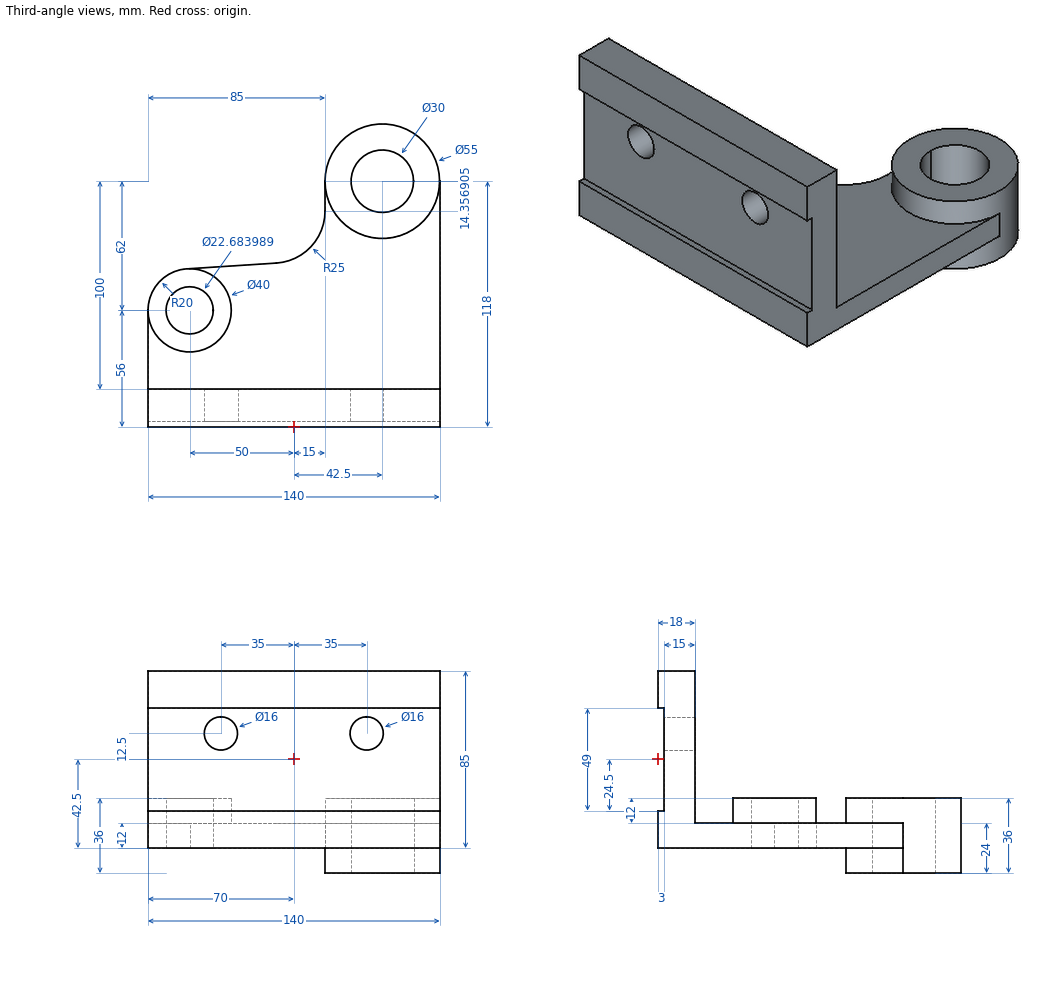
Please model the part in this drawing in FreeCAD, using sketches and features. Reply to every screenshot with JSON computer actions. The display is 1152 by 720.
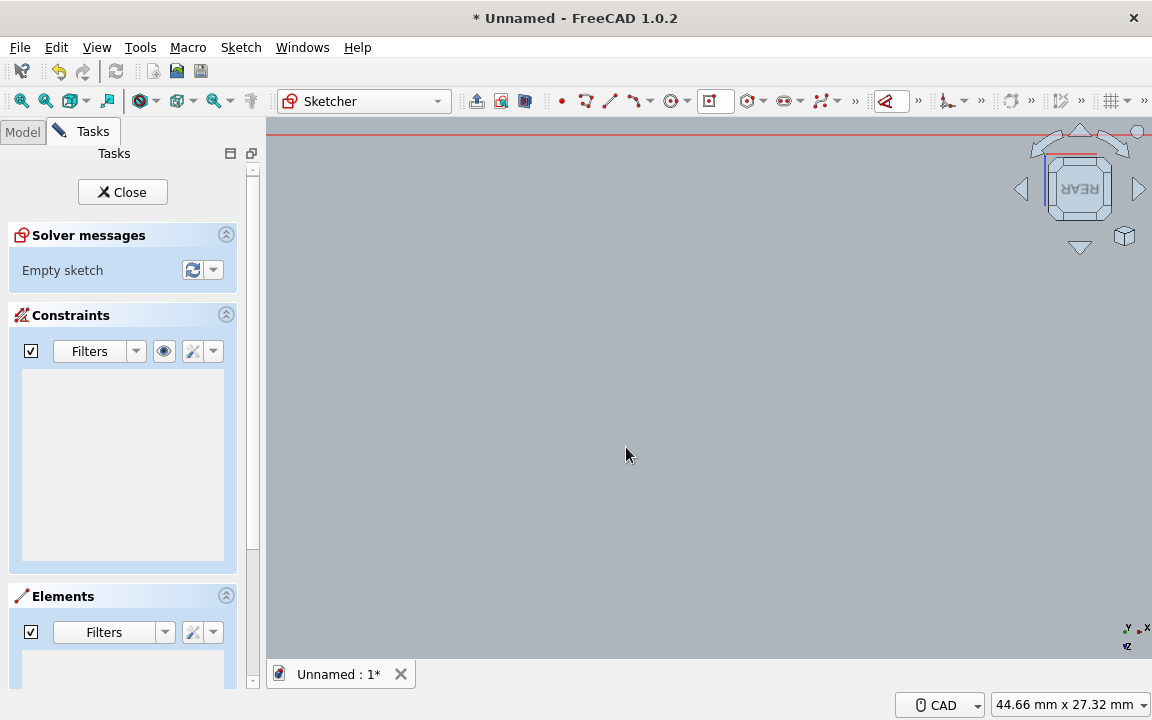
{"action": "key", "text": "g c"}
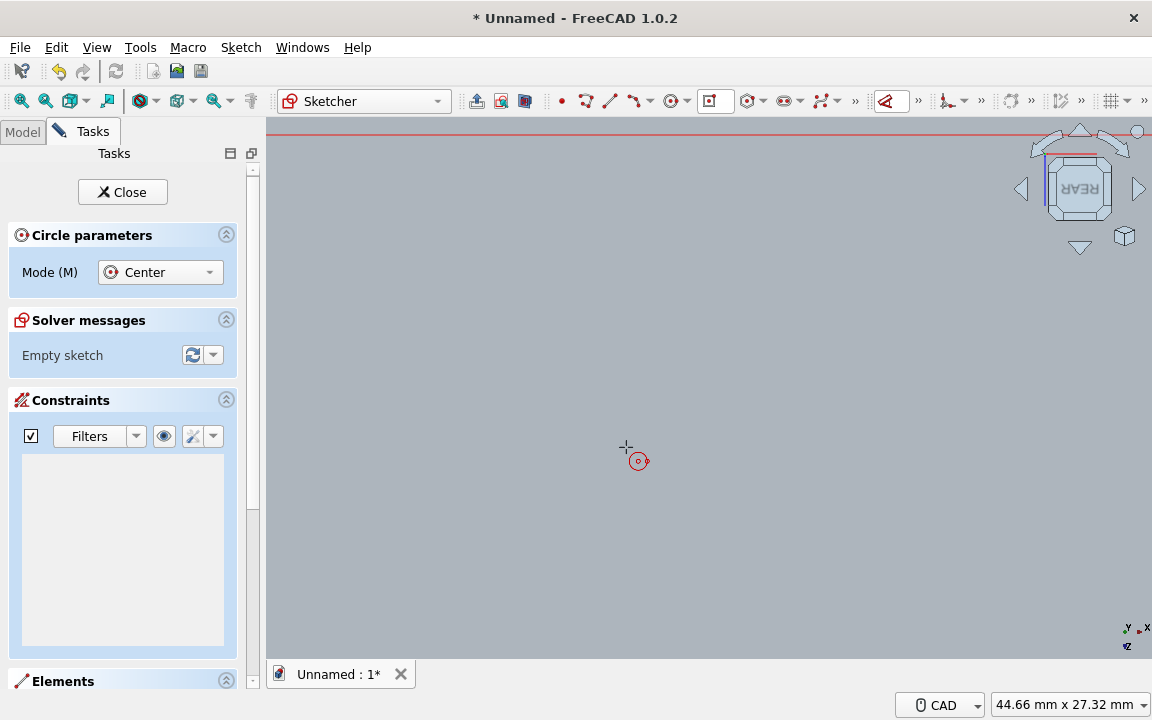
{"action": "left_click", "coordinate": [640, 383]}
{"action": "left_click", "coordinate": [753, 271]}
{"action": "key", "text": "Escape"}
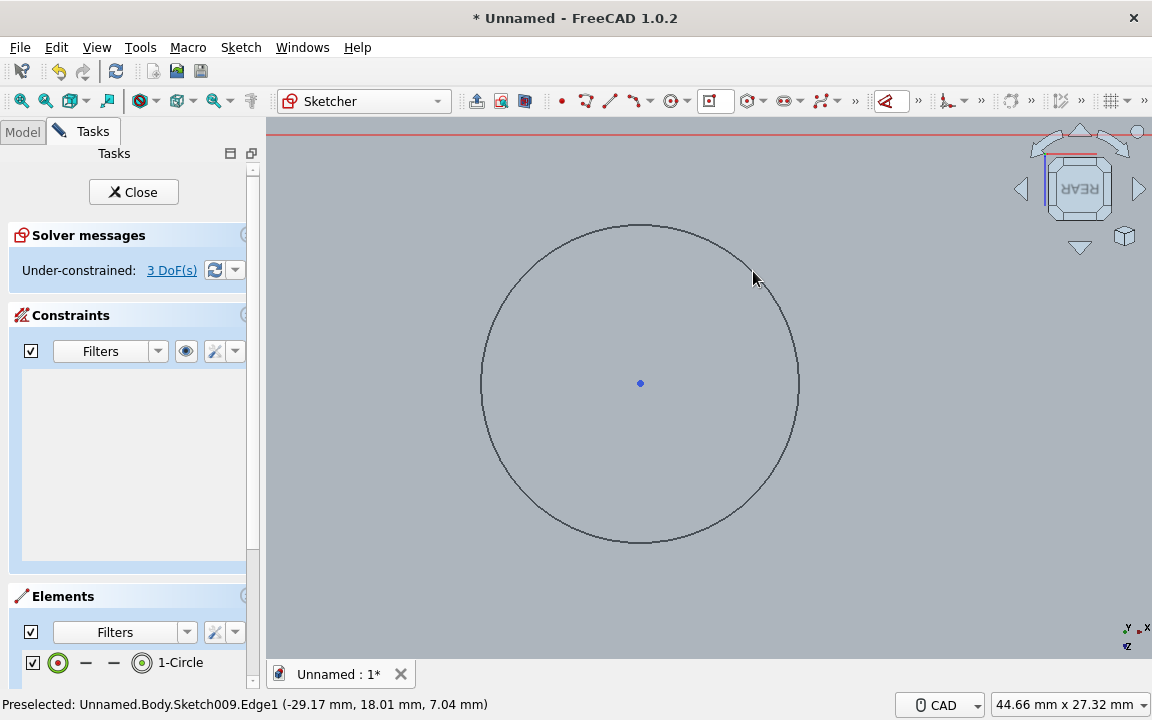
{"action": "left_click", "coordinate": [752, 271]}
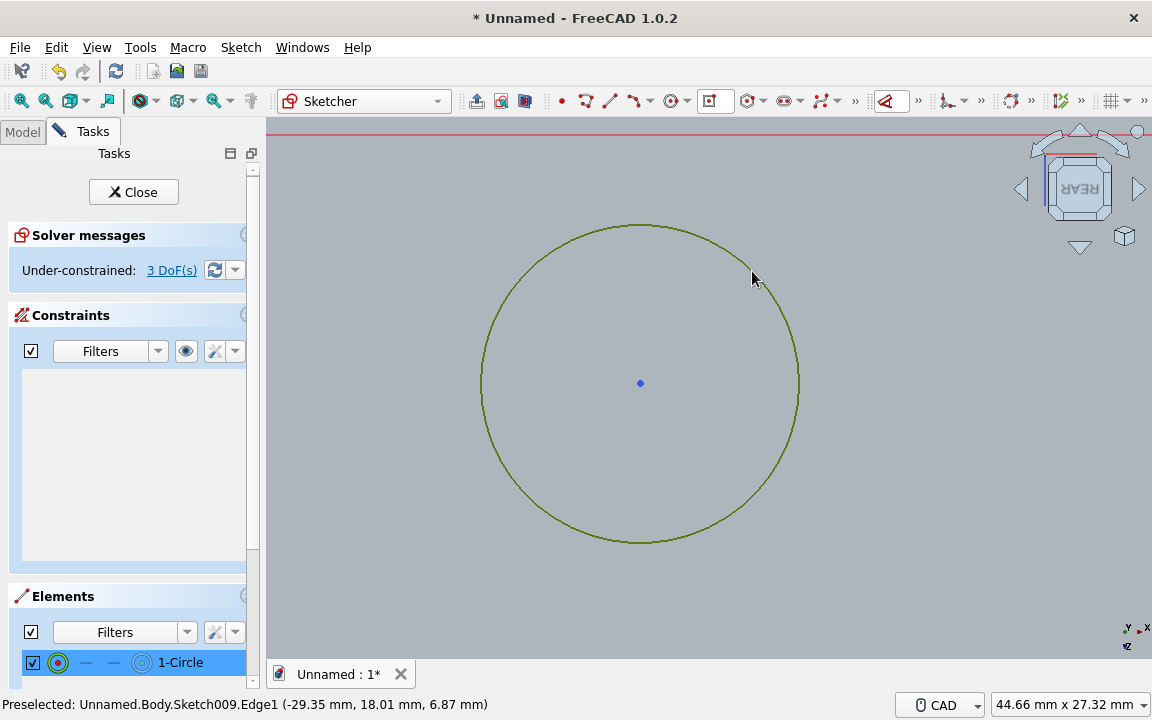
{"action": "key", "text": "k o"}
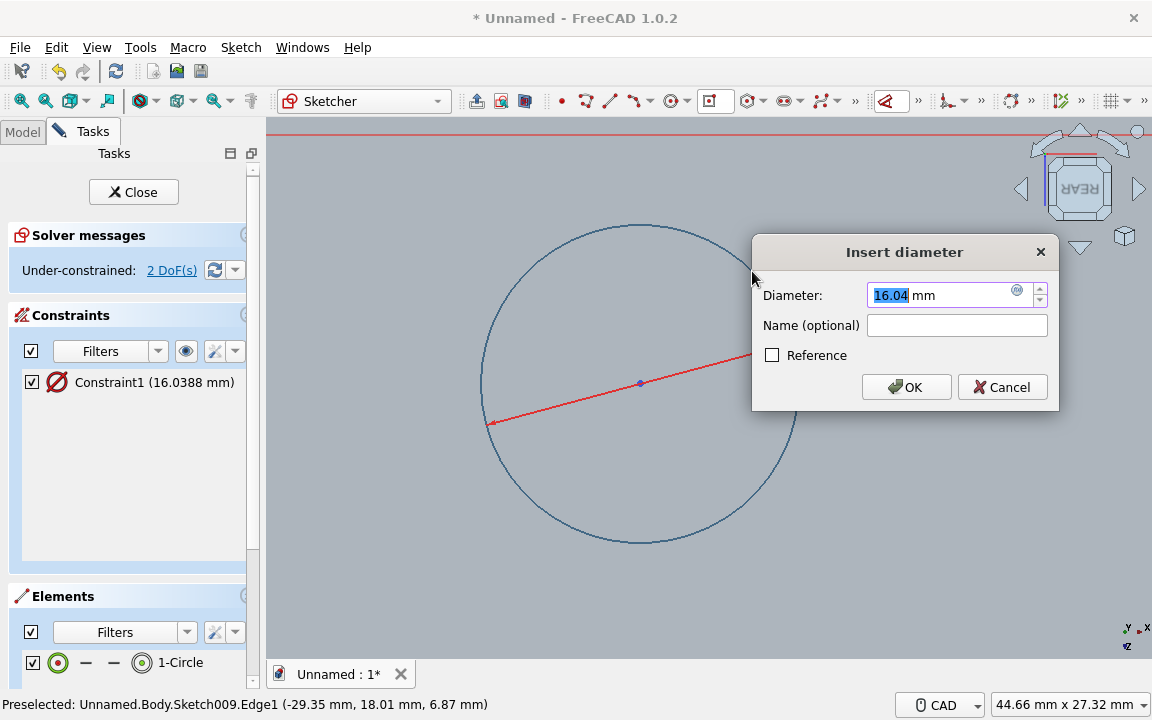
{"action": "type", "text": "16"}
{"action": "key", "text": "Return"}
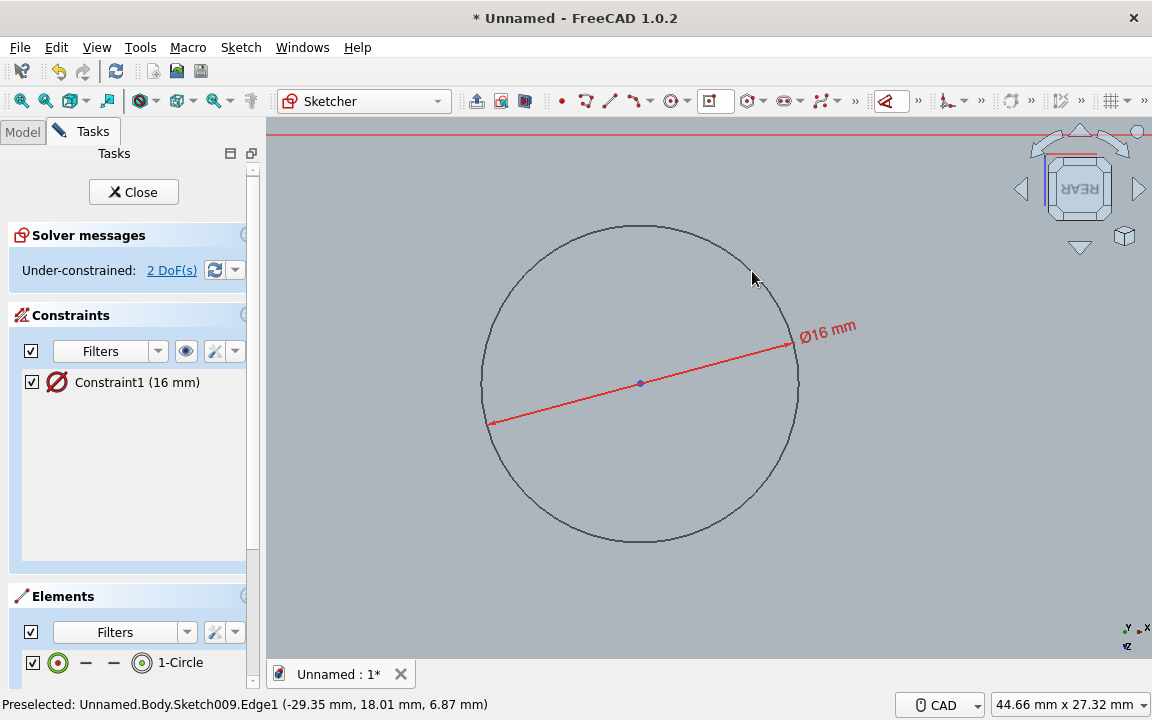
{"action": "left_click", "coordinate": [640, 384]}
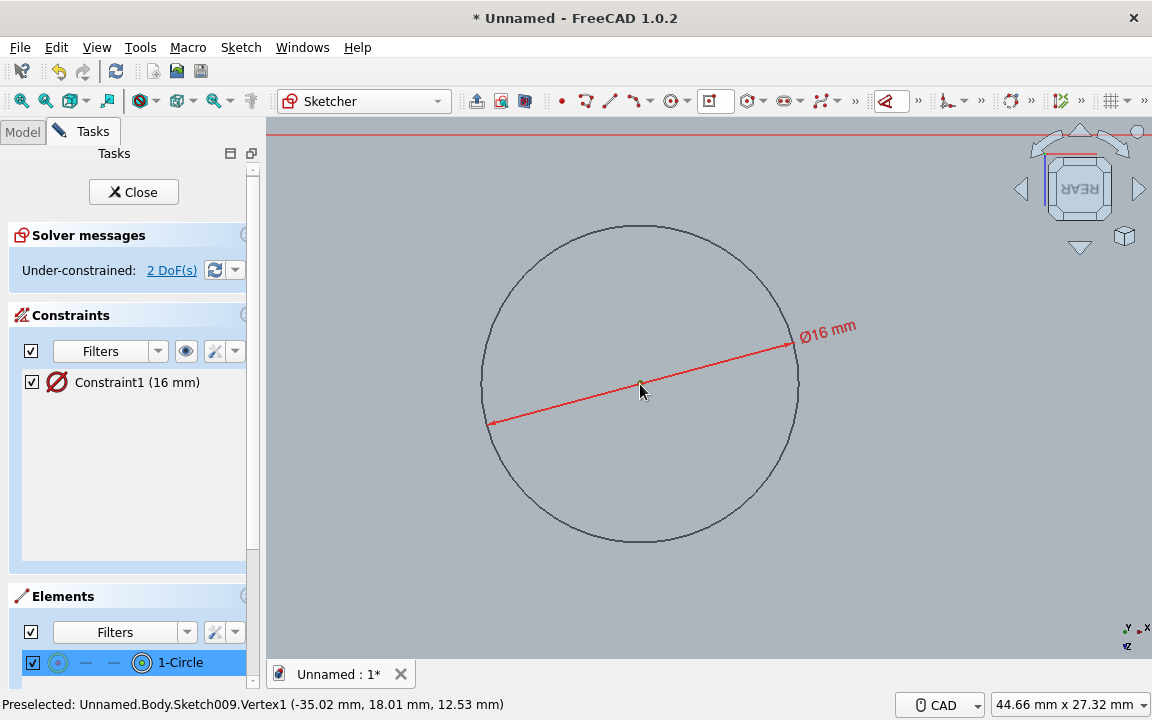
{"action": "key", "text": "l"}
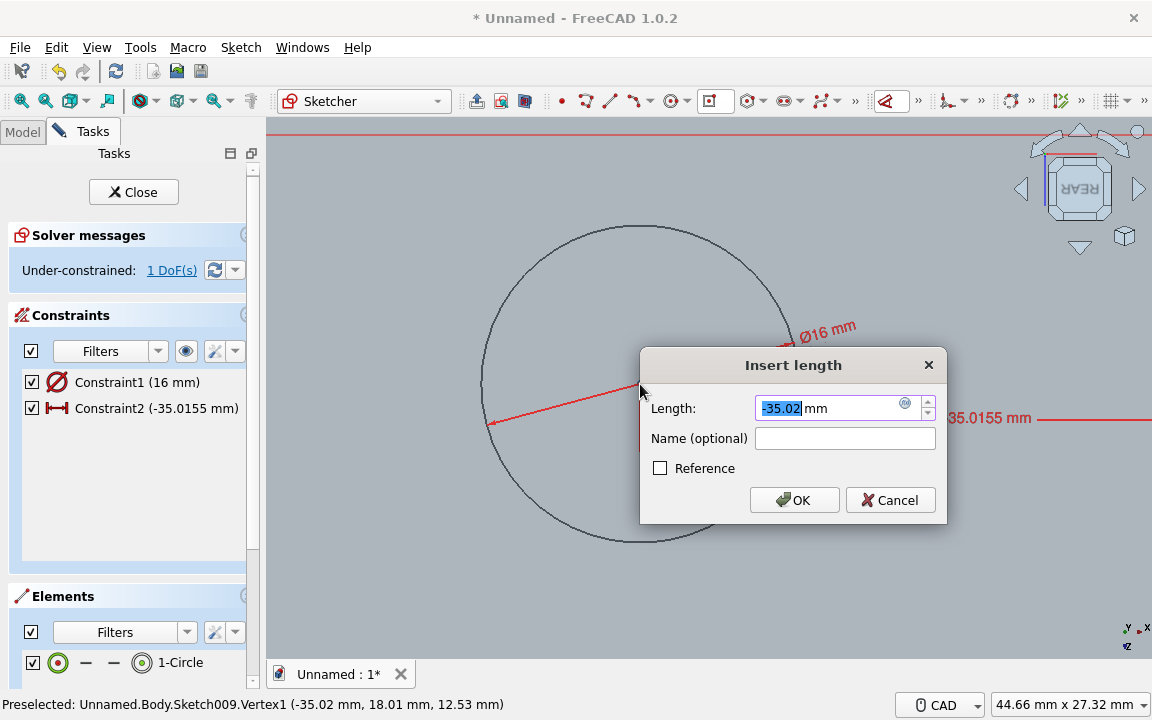
{"action": "type", "text": "-35"}
{"action": "key", "text": "Return"}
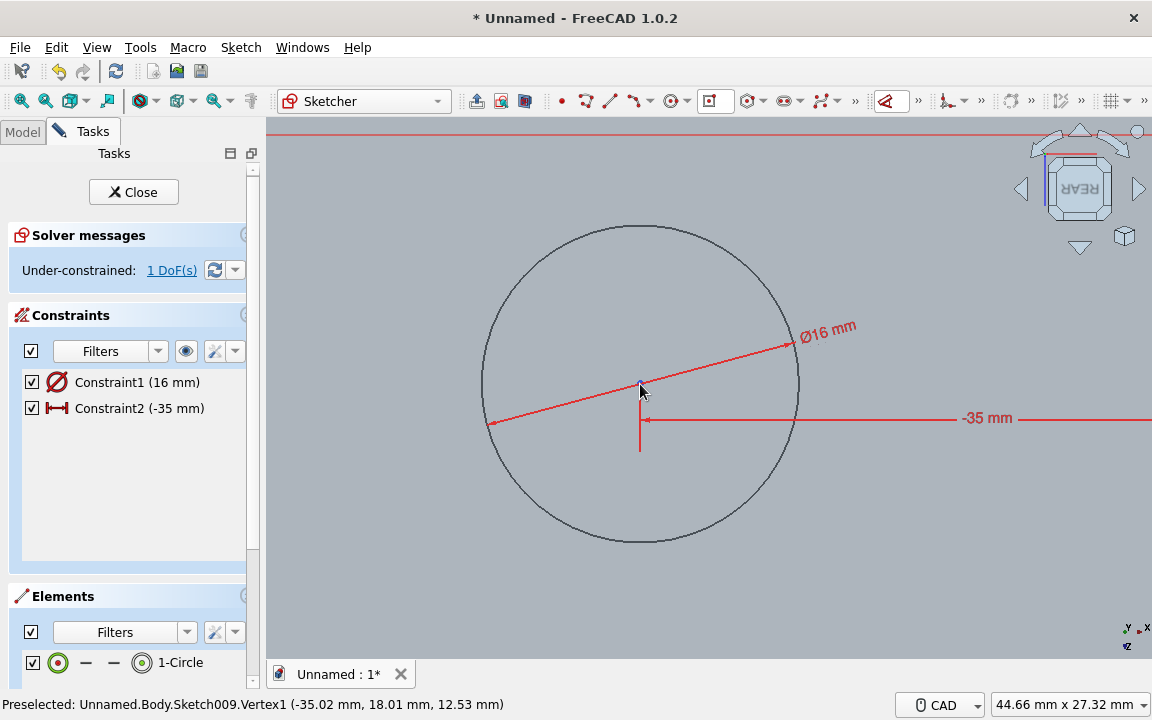
{"action": "left_click", "coordinate": [640, 384]}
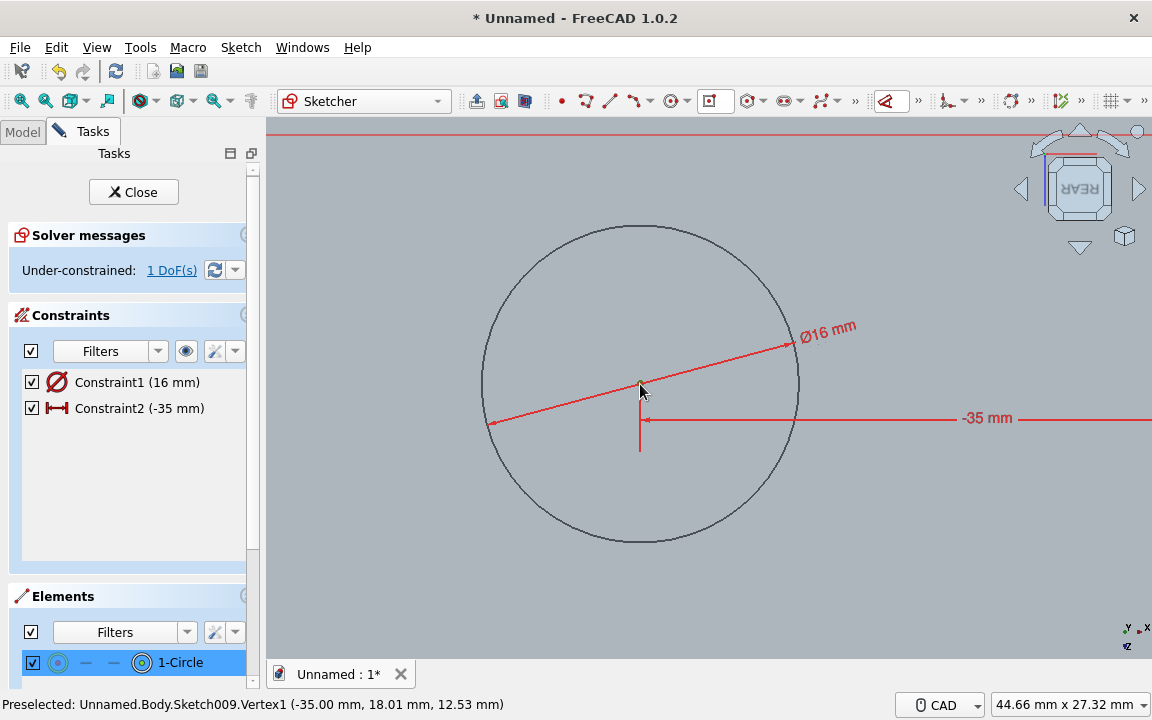
{"action": "key", "text": "i"}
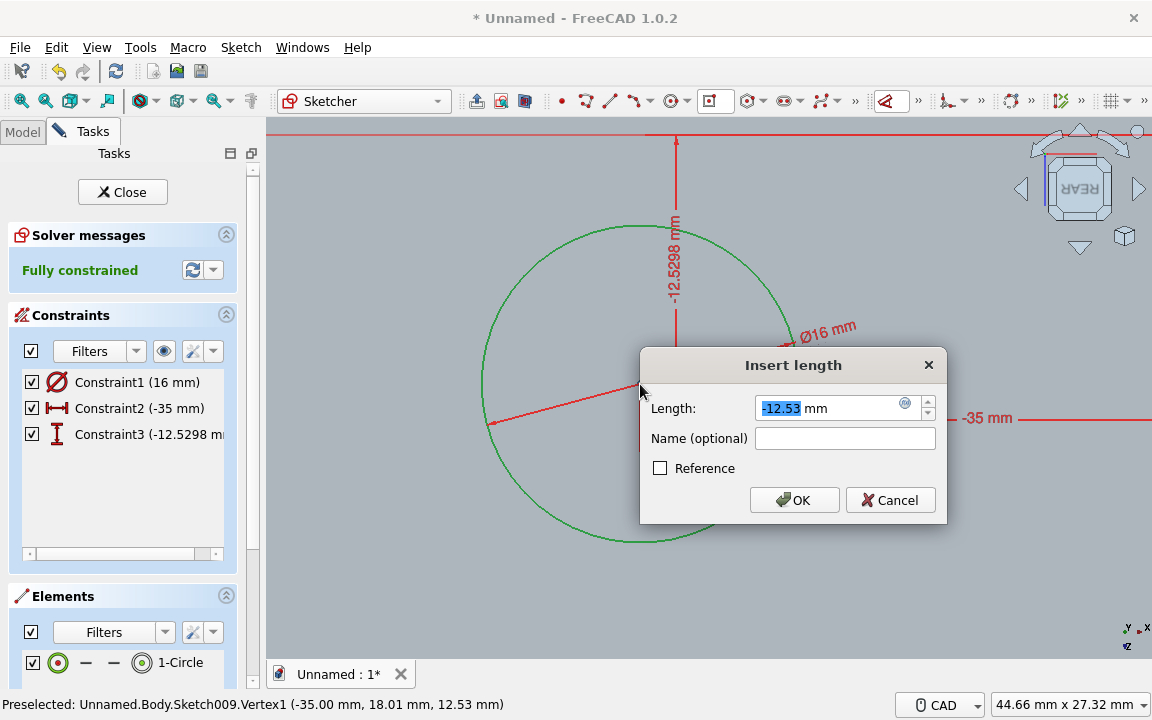
{"action": "type", "text": "-12.5"}
{"action": "key", "text": "Return"}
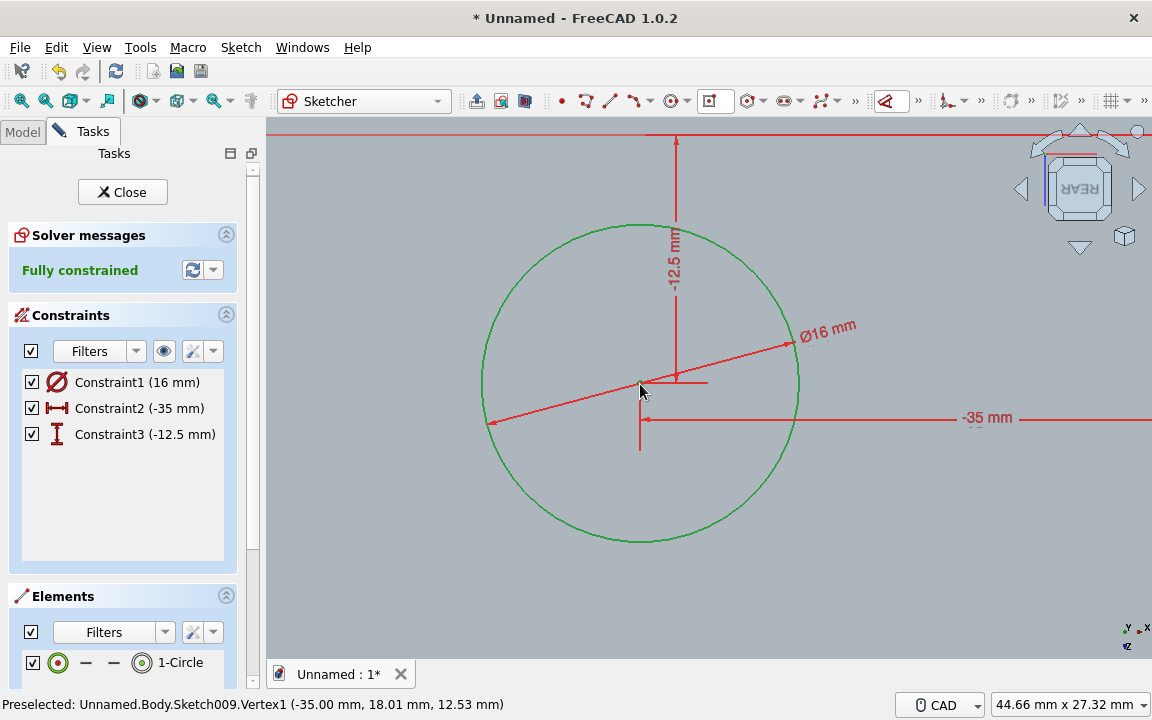
{"action": "left_click", "coordinate": [123, 192]}